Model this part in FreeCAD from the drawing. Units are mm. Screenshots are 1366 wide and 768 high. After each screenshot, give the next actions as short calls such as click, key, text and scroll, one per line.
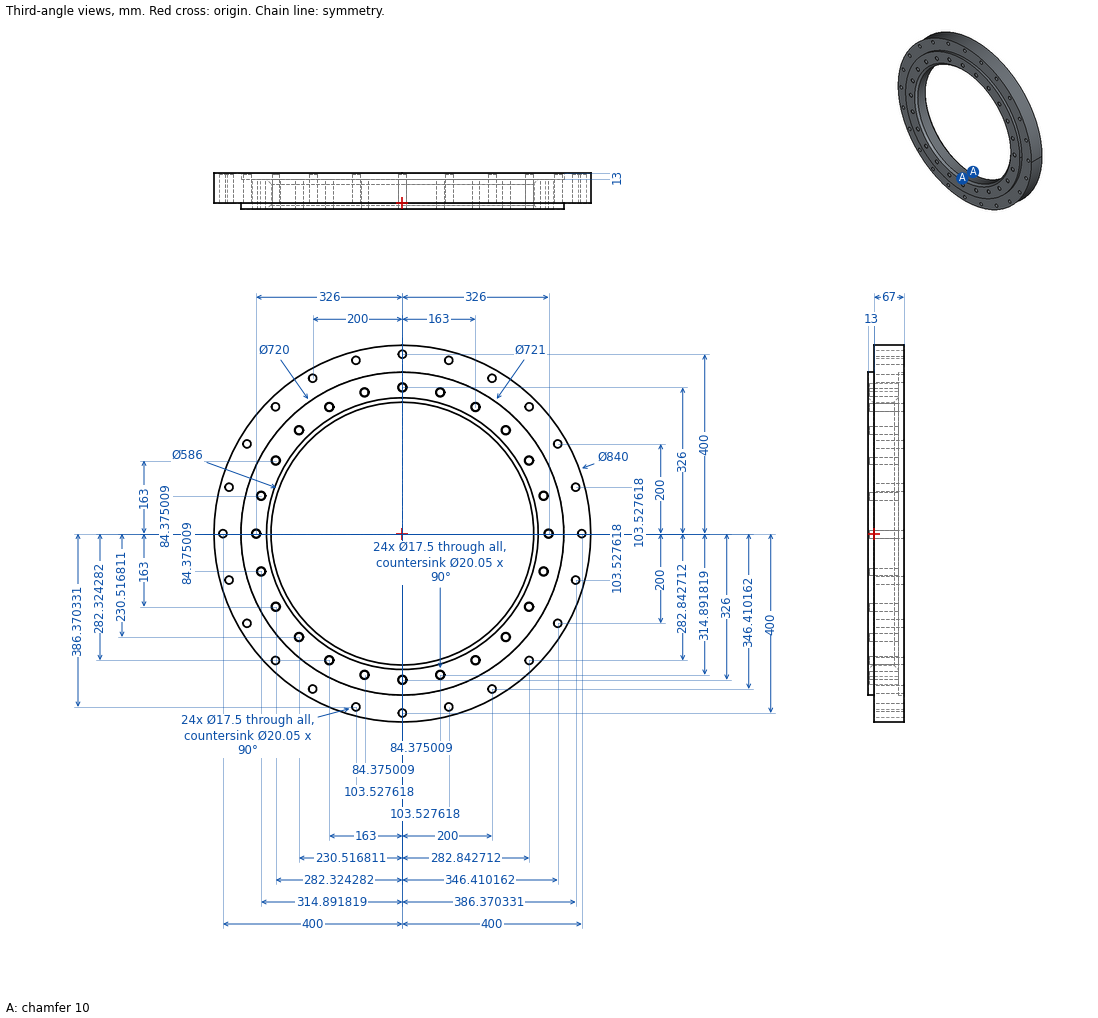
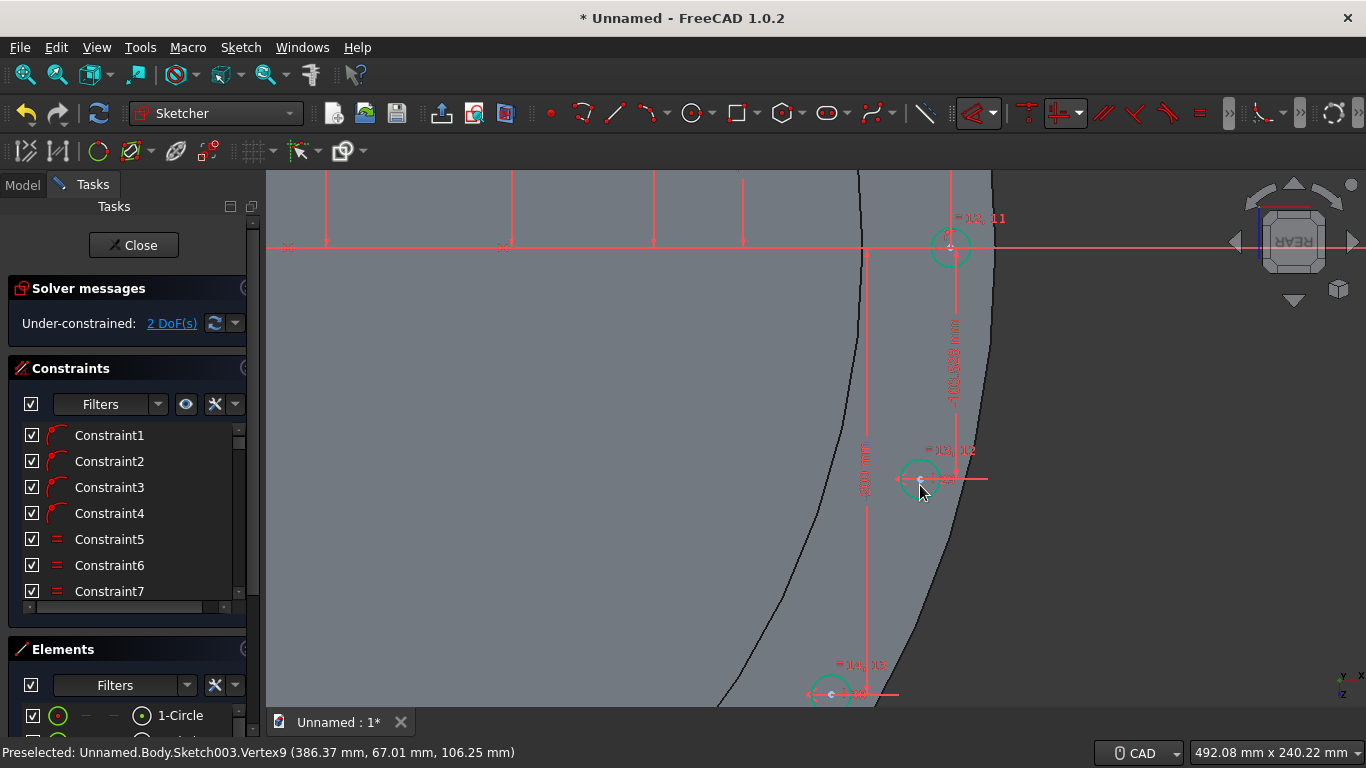
scroll(922, 487, down, 8)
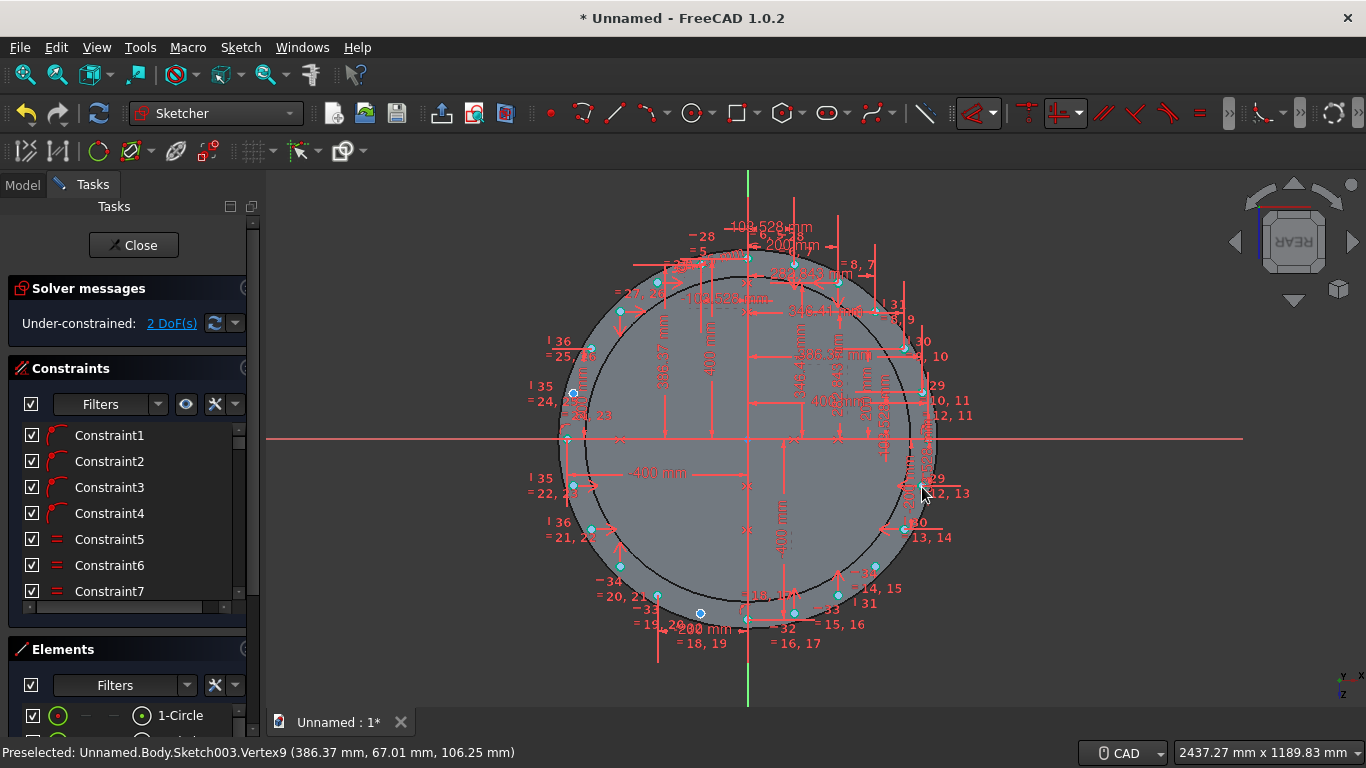
click(701, 614)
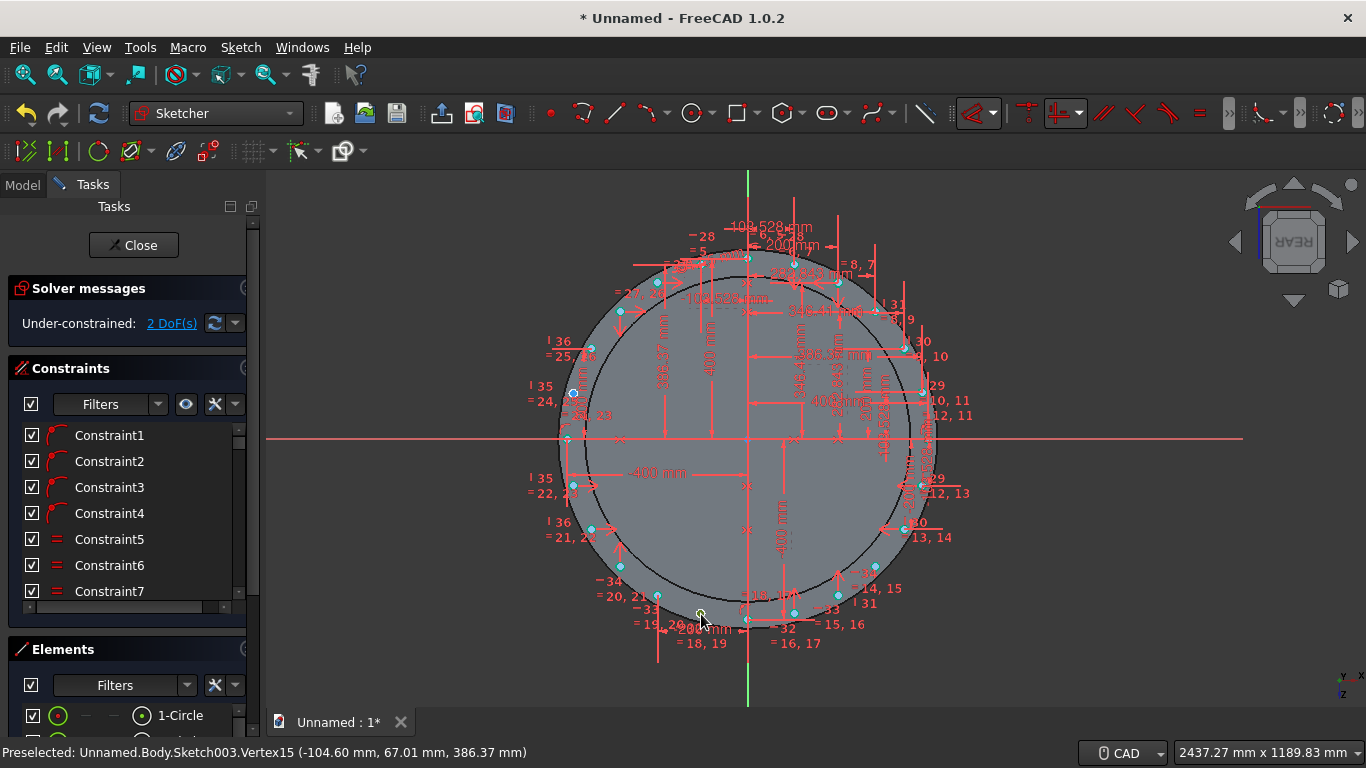
key(l)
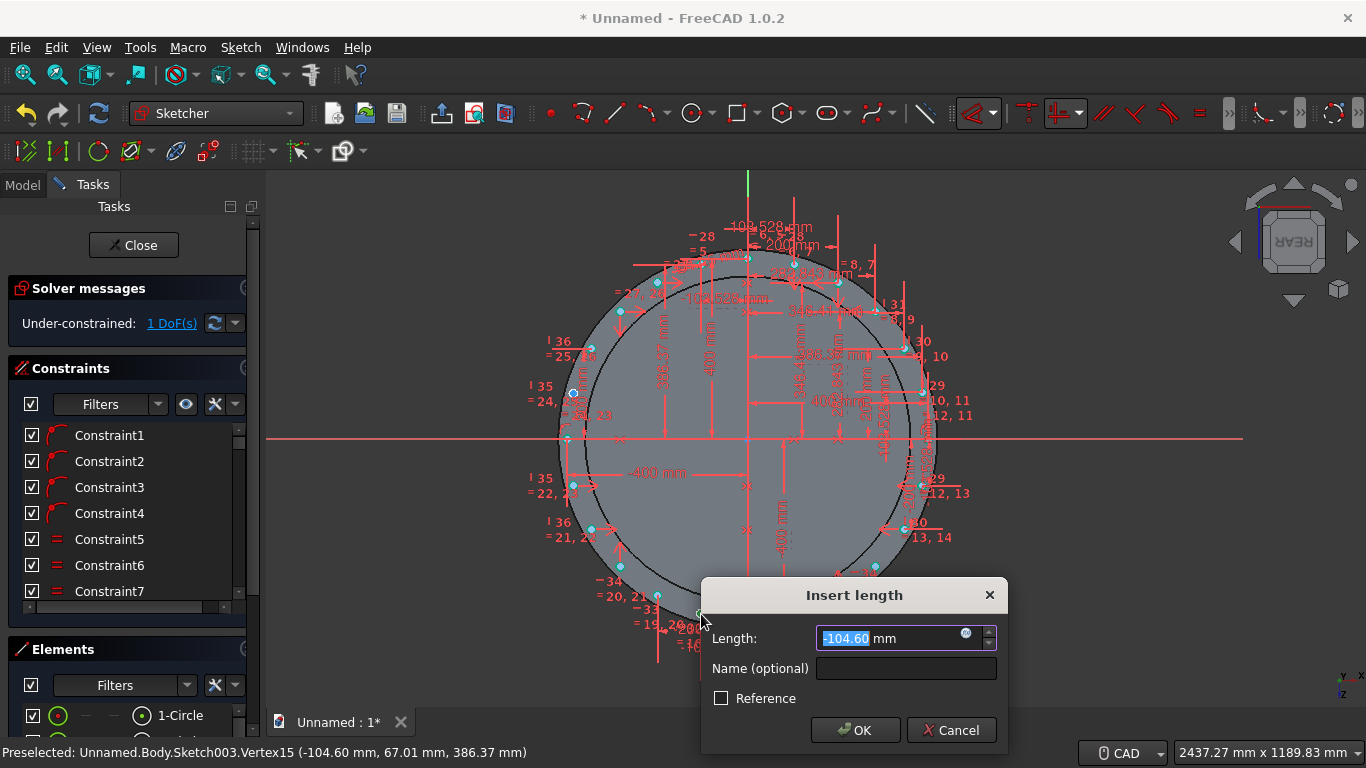
text(-103.527618)
key(Return)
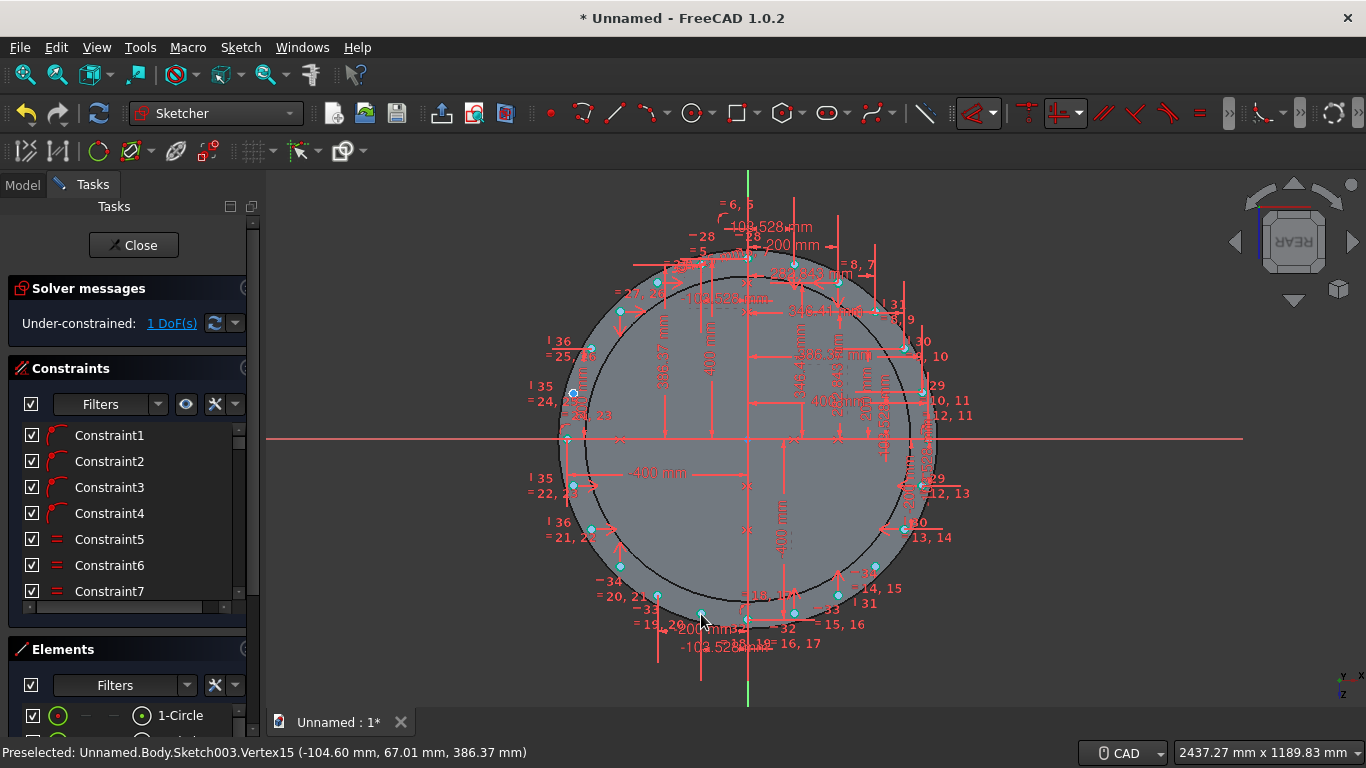
scroll(573, 394, up, 4)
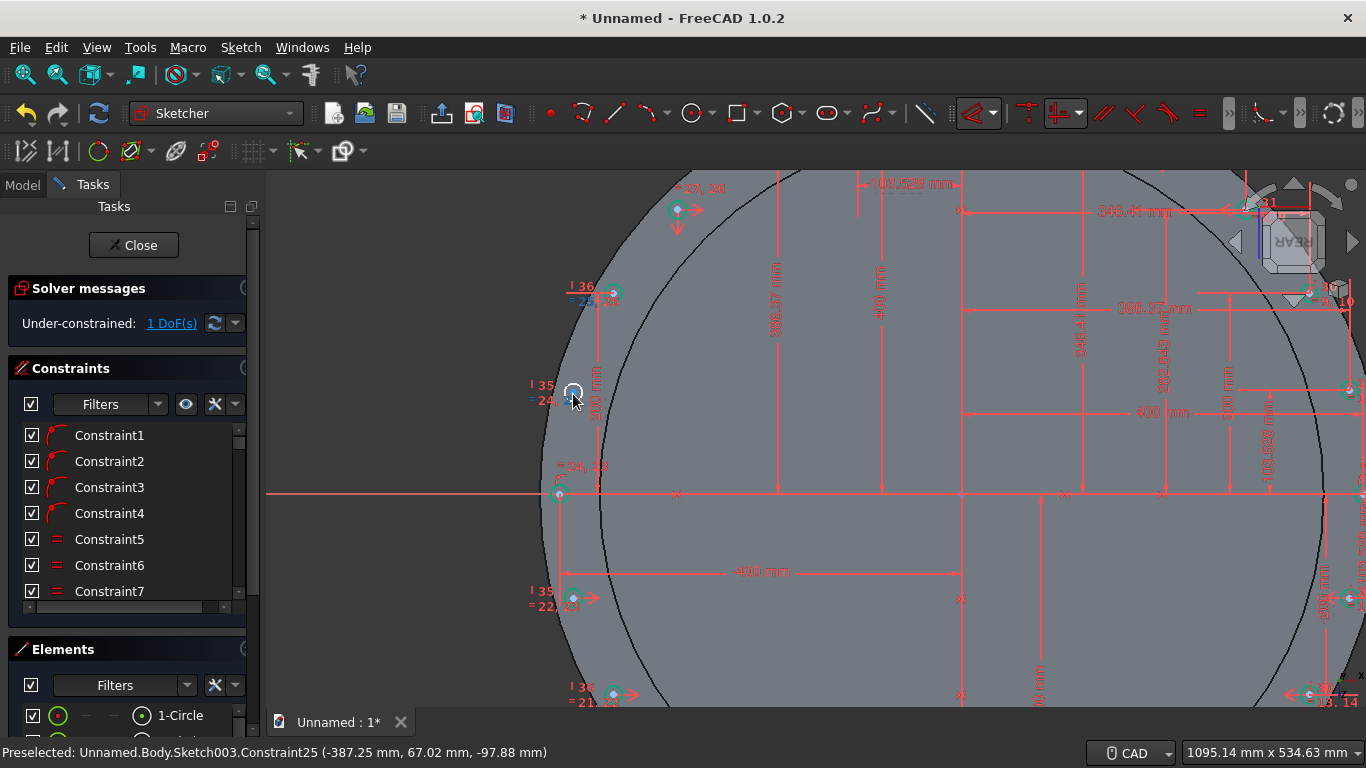
scroll(574, 392, up, 4)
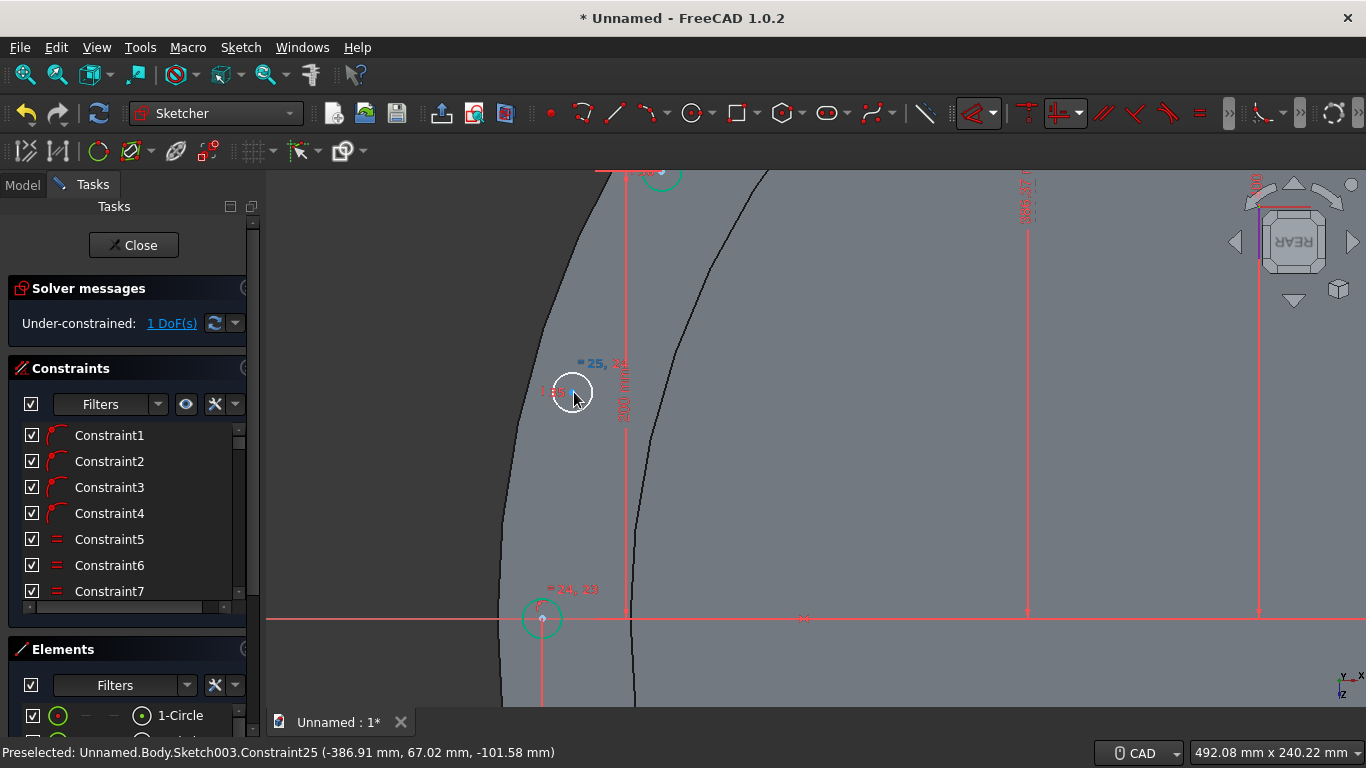
click(573, 392)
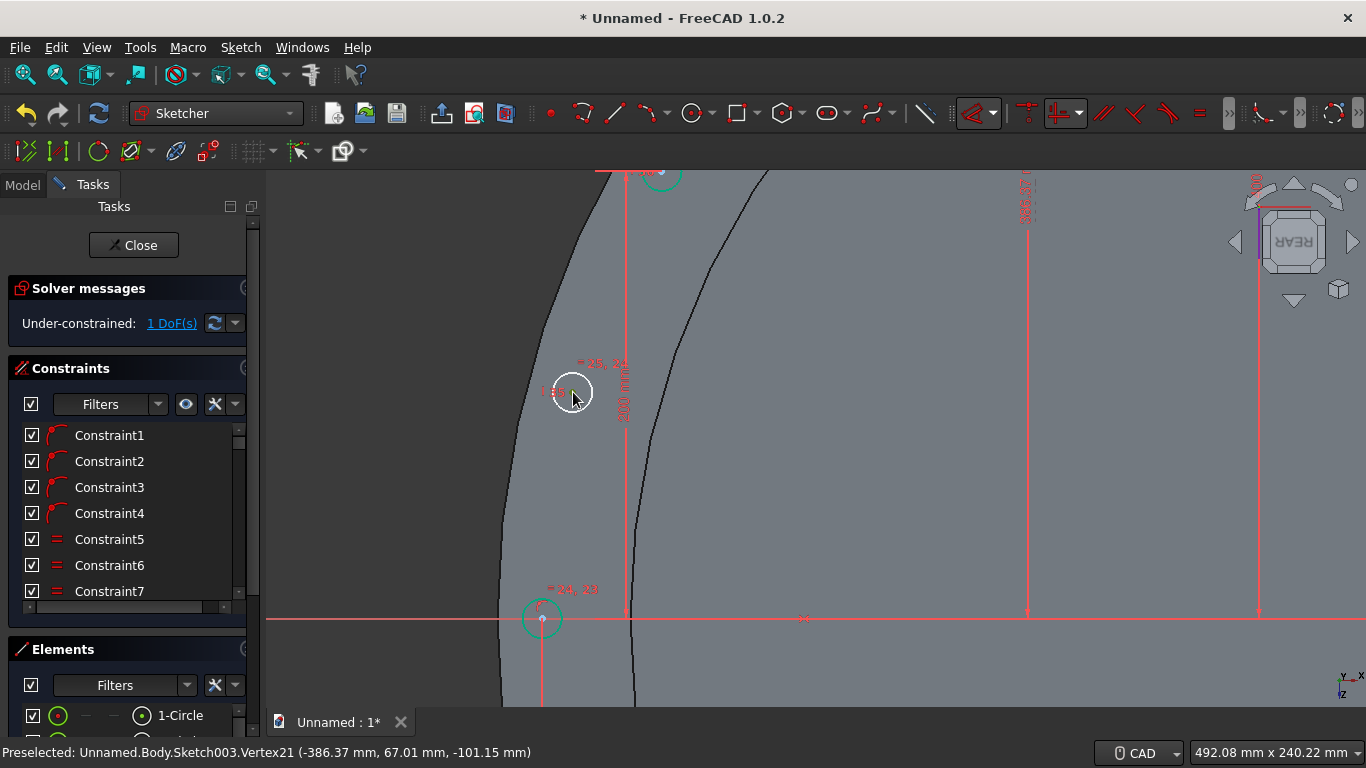
key(i)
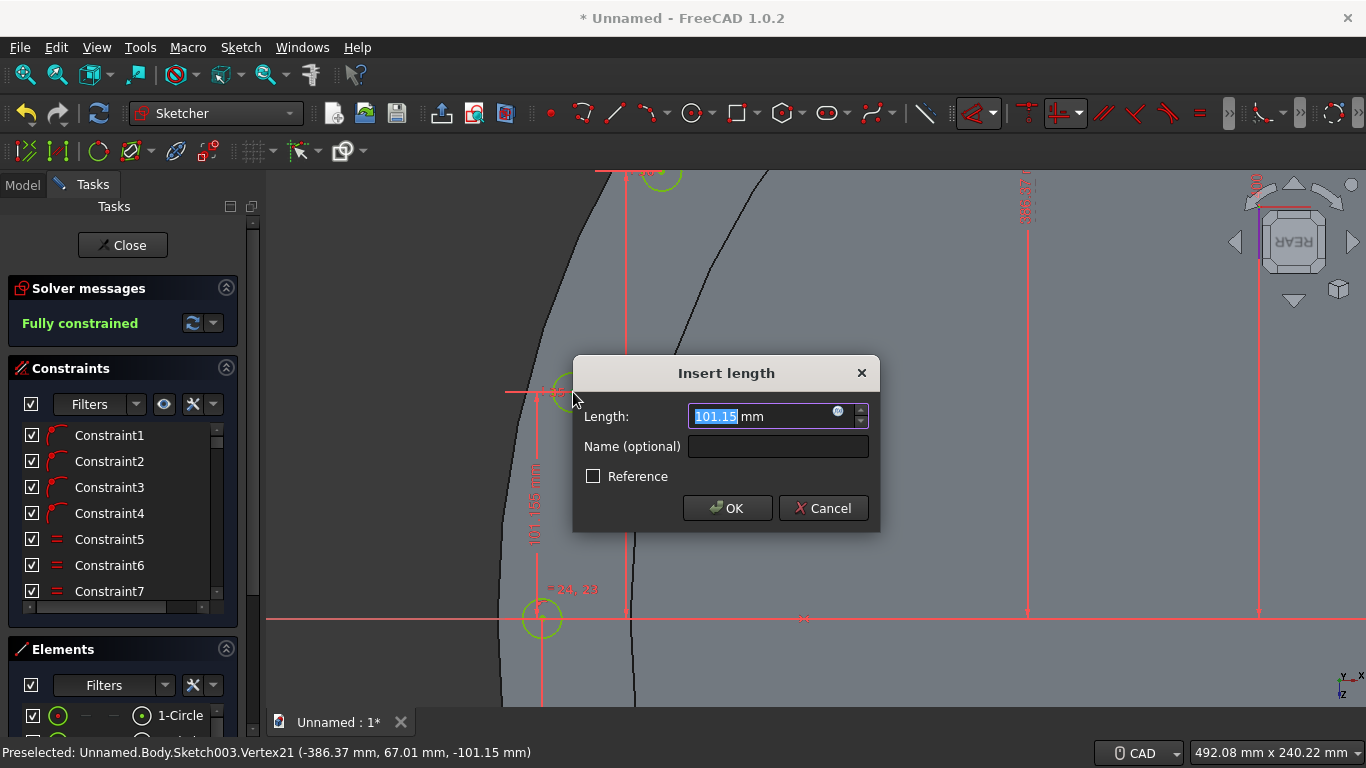
text(103.527618)
key(Return)